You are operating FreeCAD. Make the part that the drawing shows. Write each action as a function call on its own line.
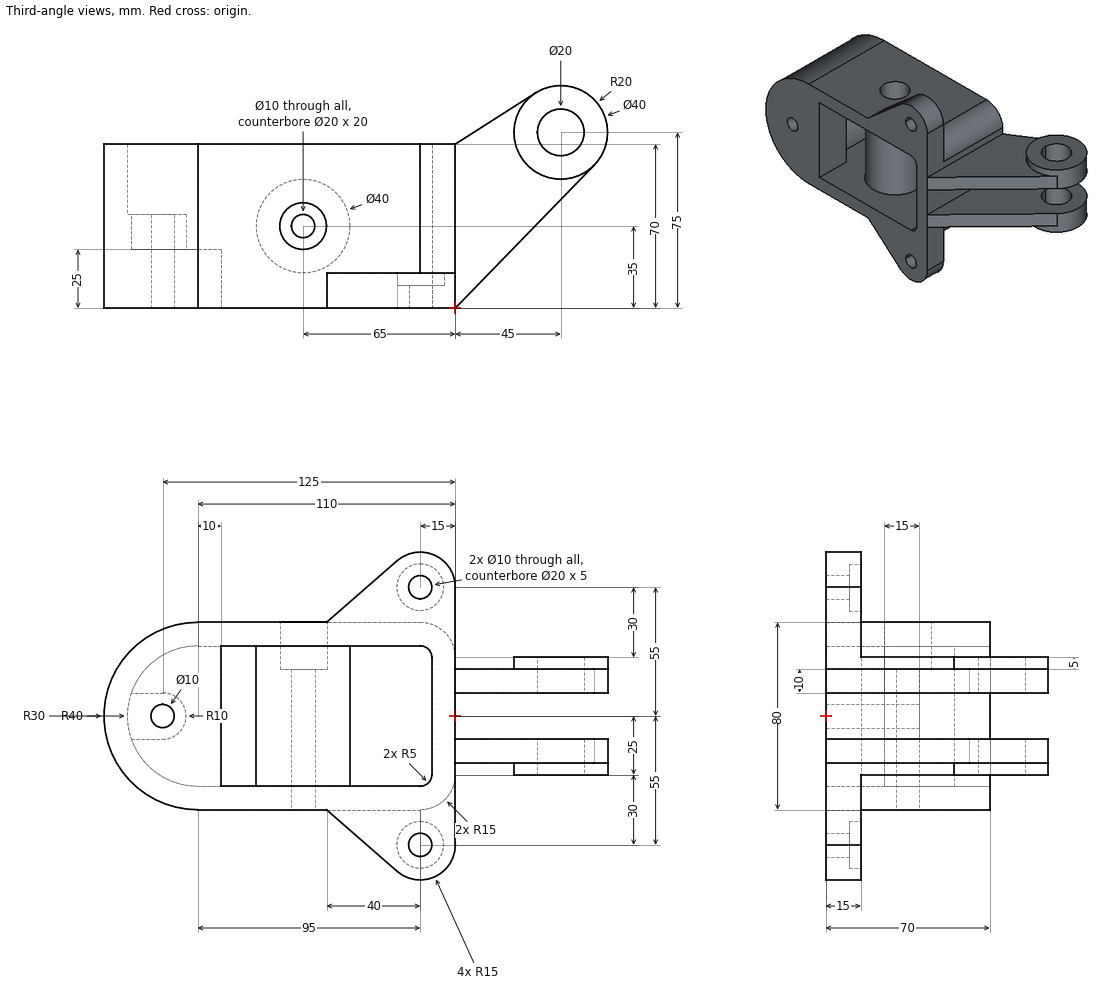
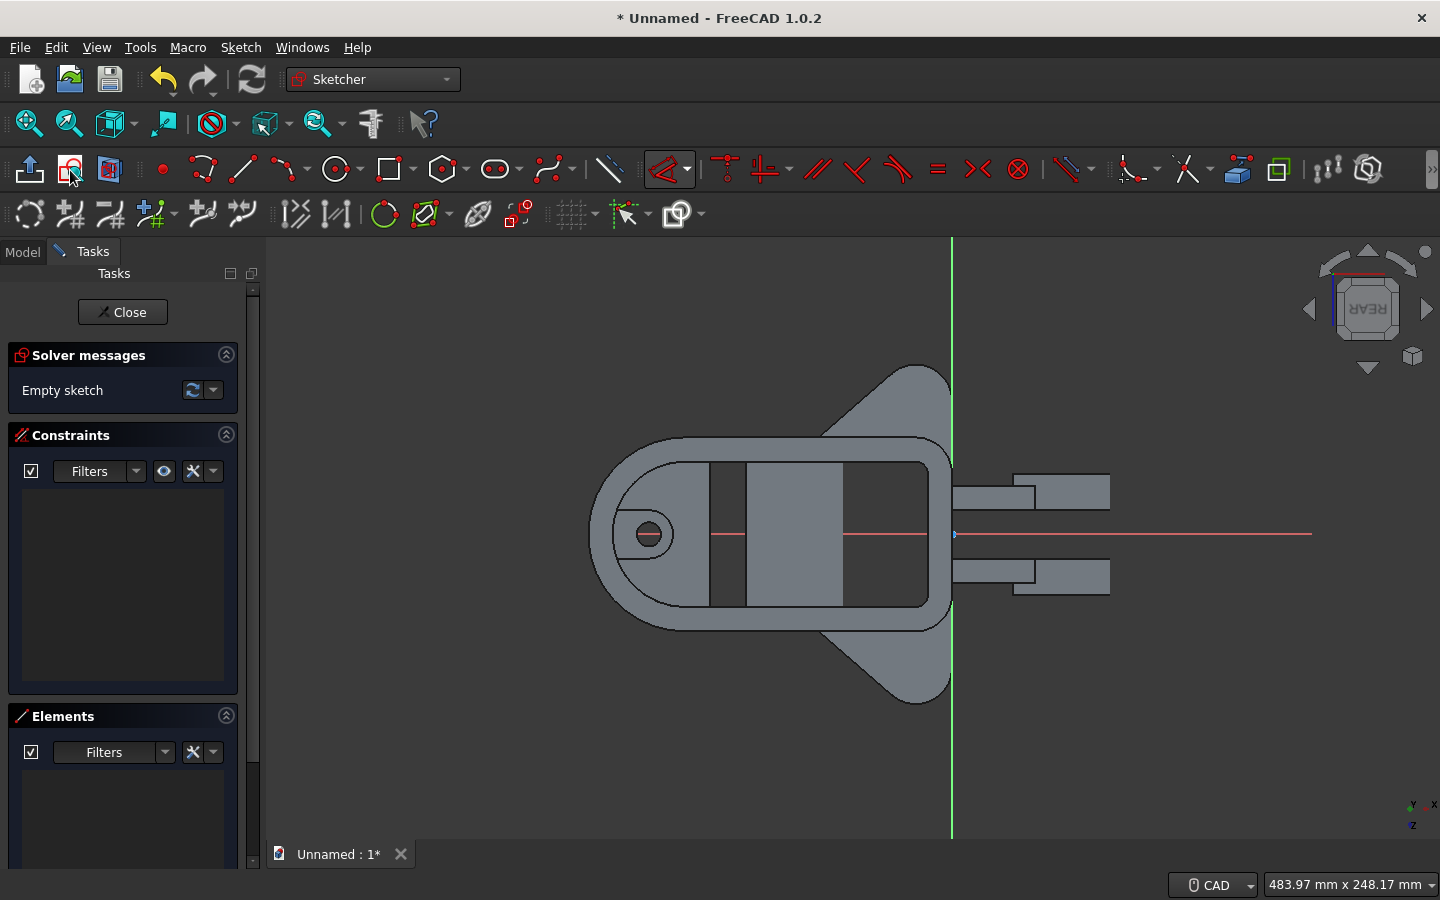
key(q)
key(s)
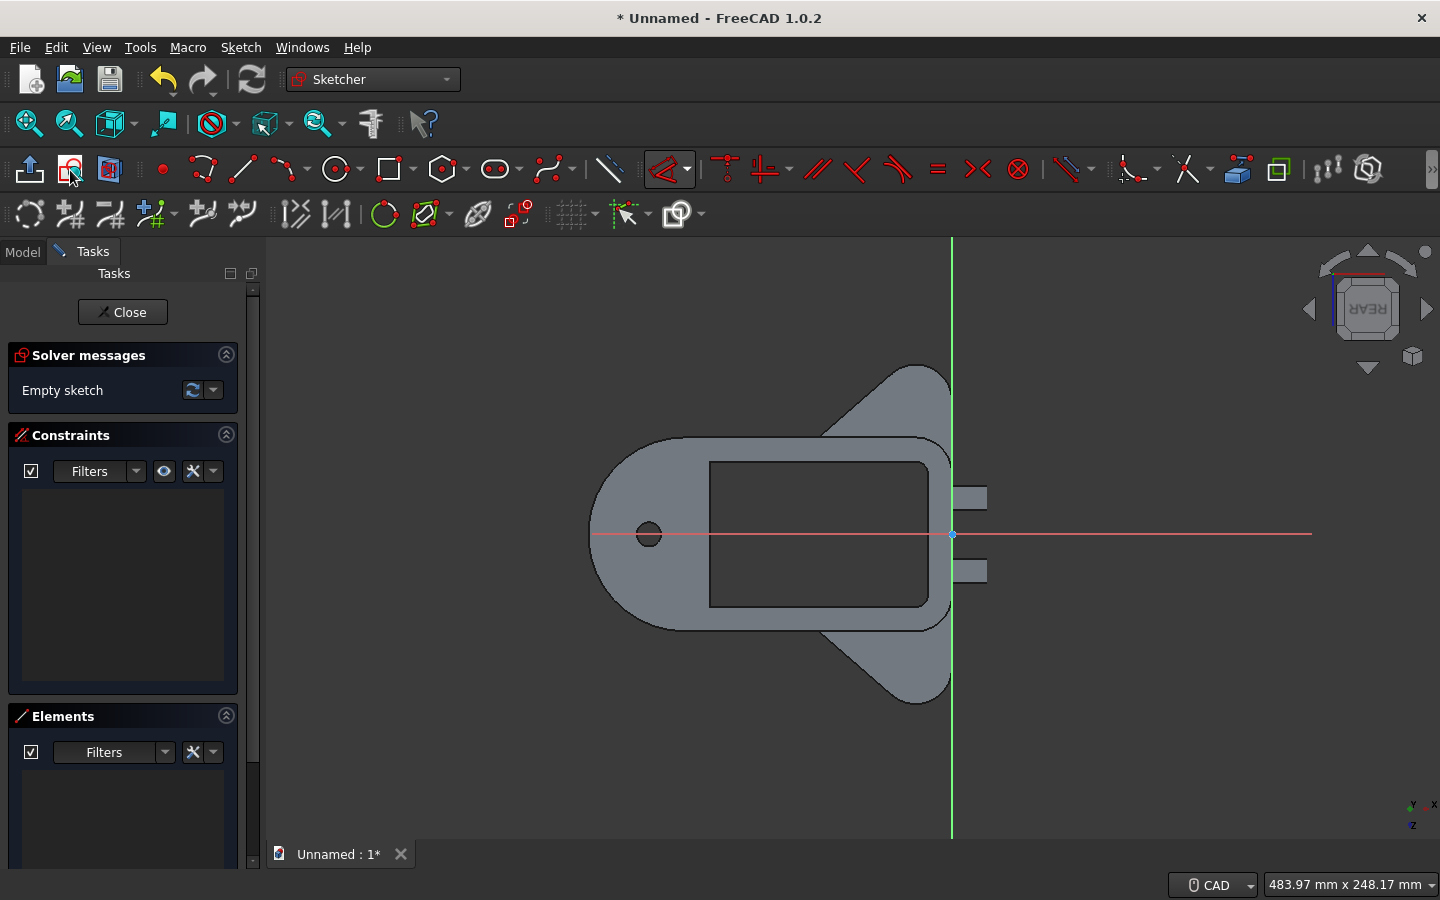
key(g)
key(c)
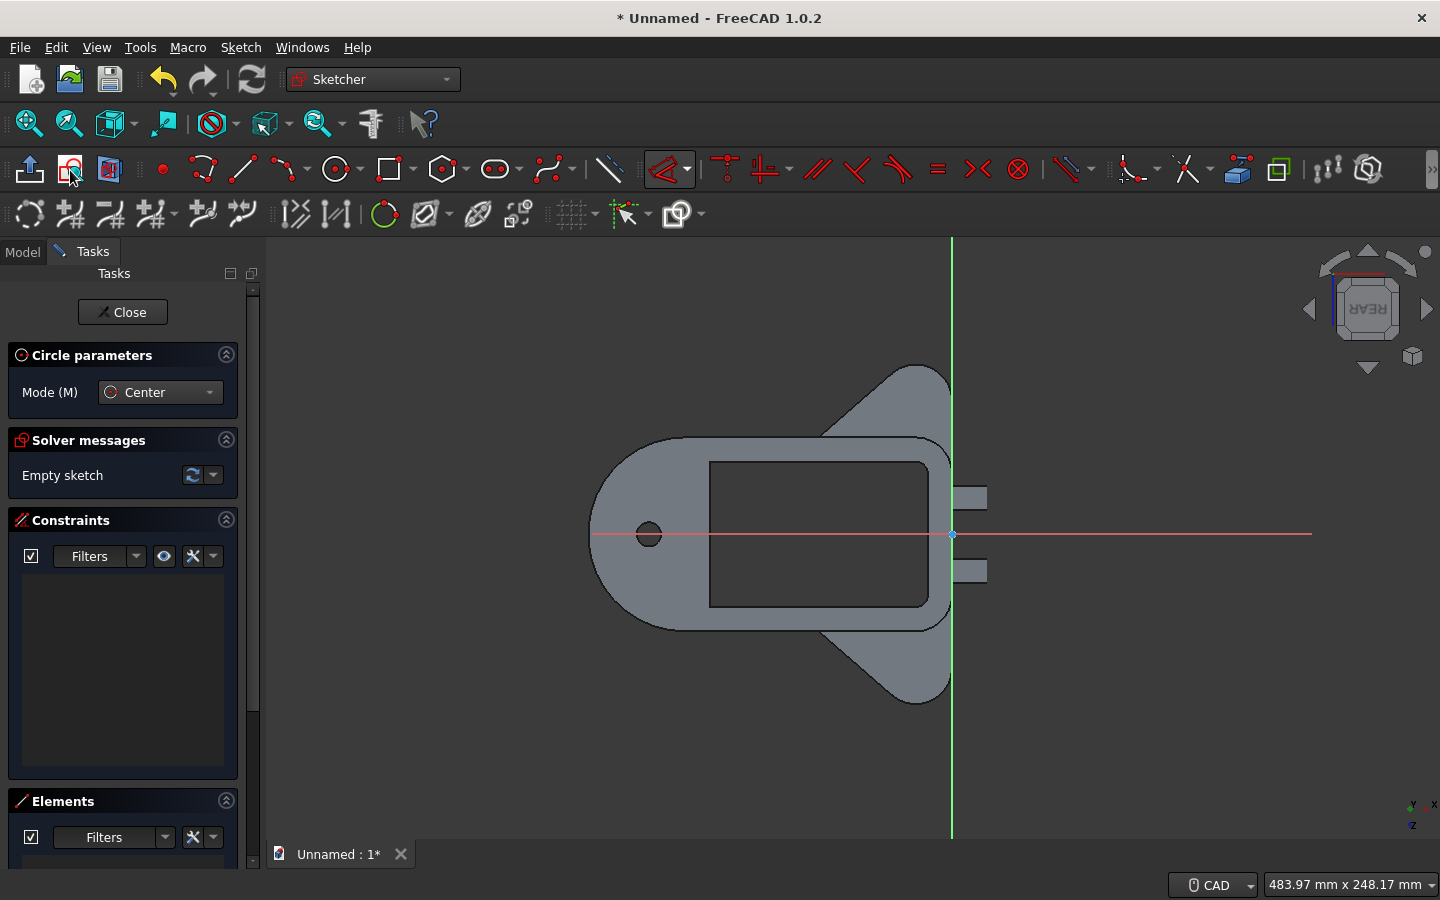
scroll(916, 668, up, 4)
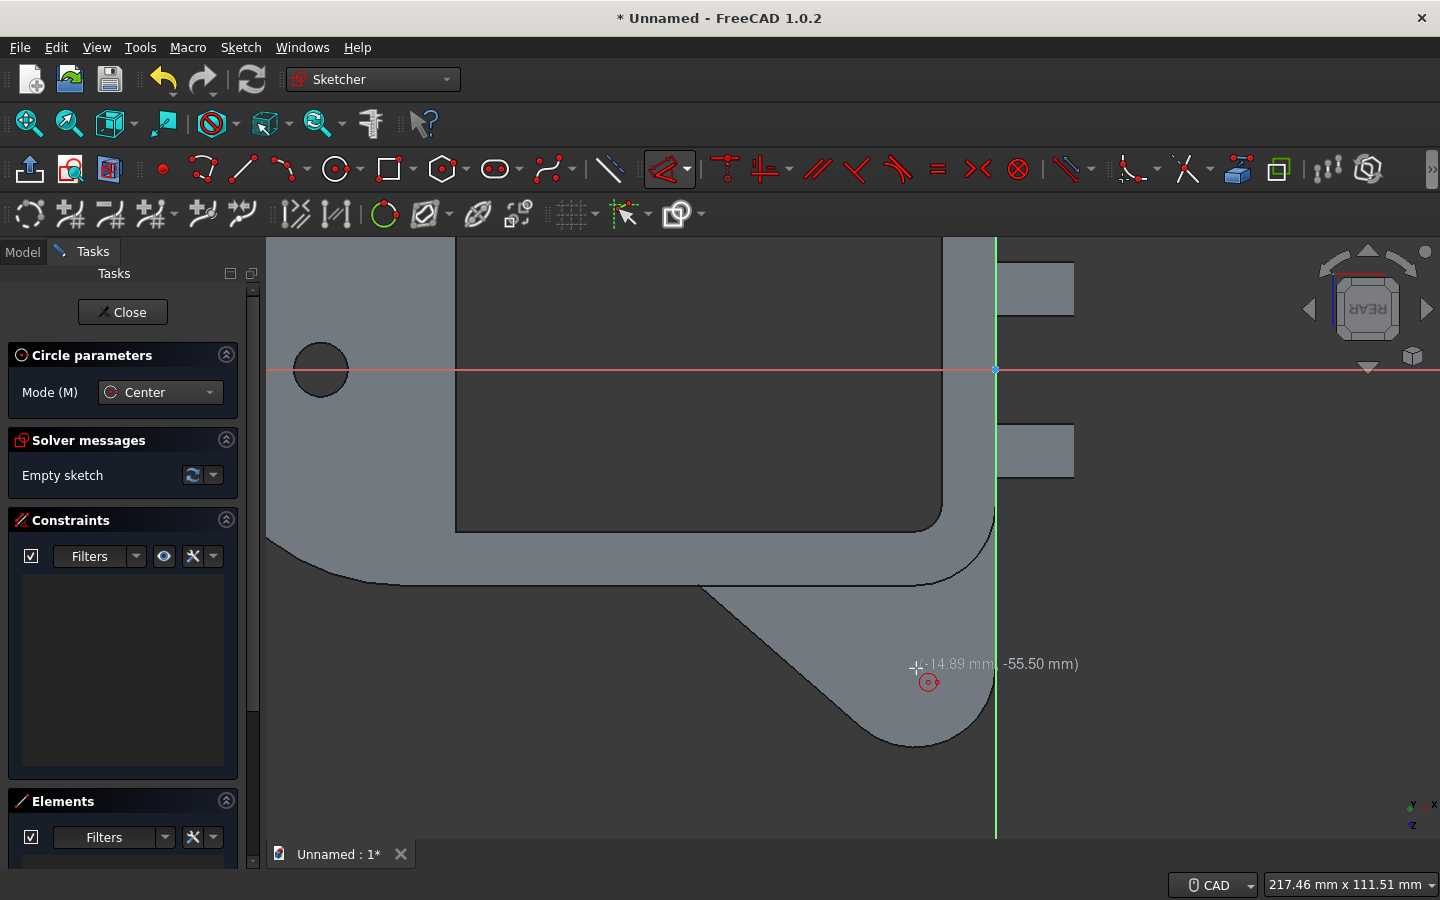
click(915, 667)
move(934, 648)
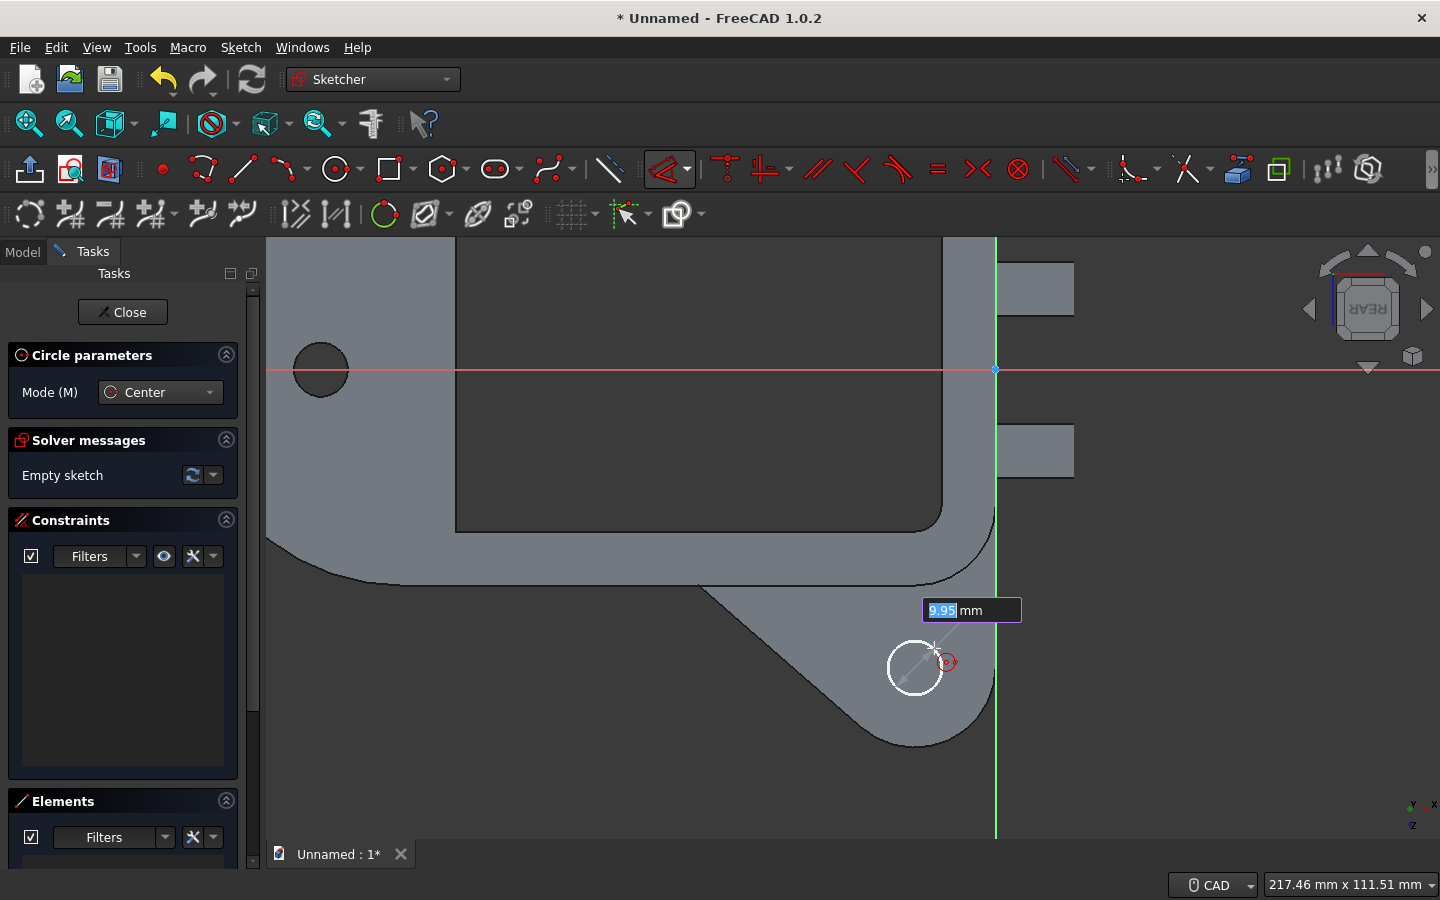
text(10)
key(Return)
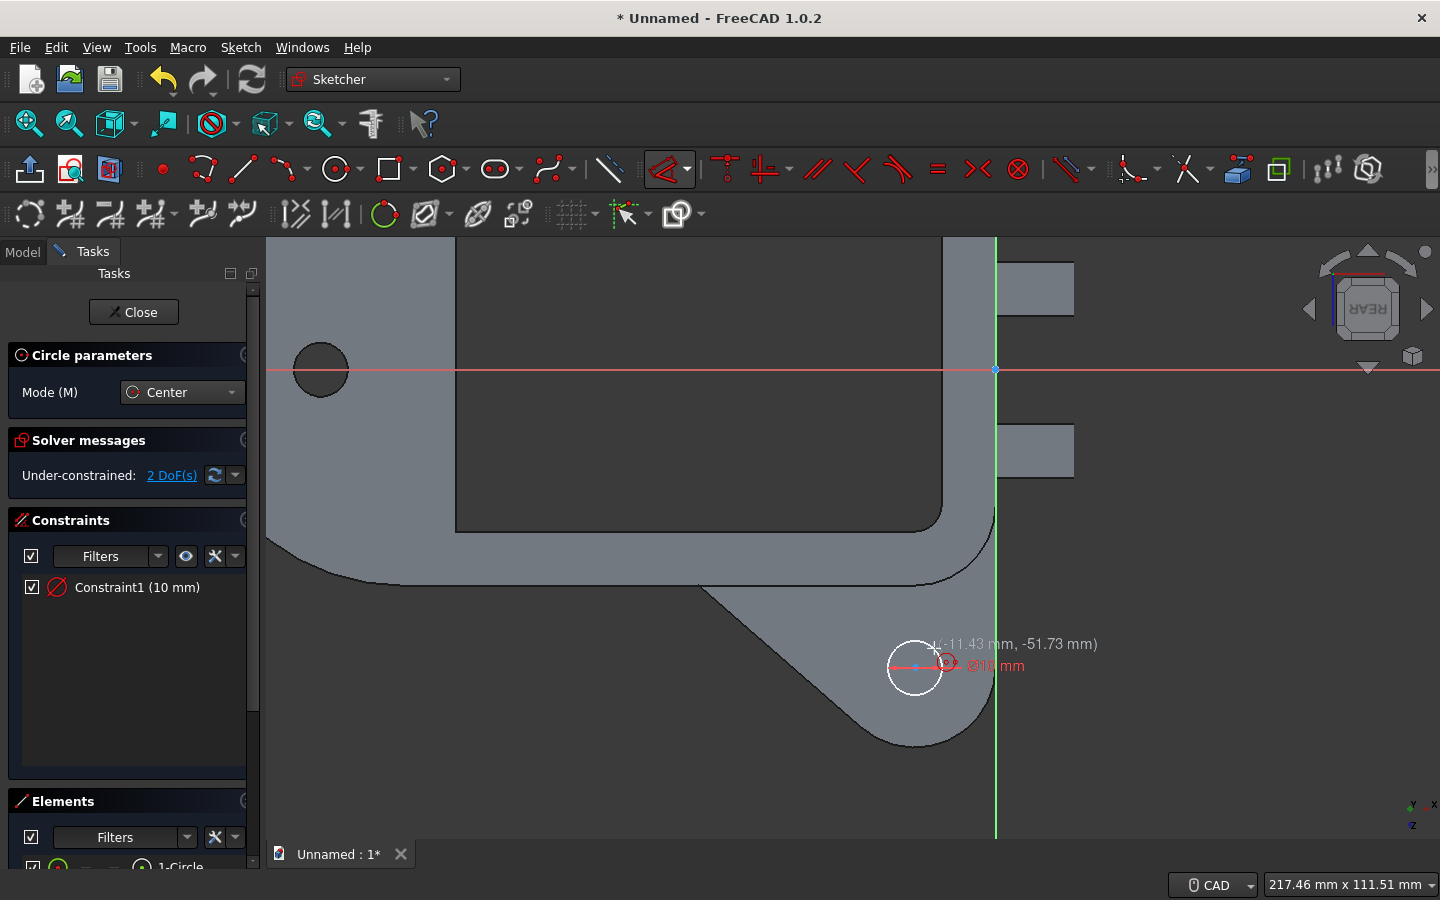
scroll(593, 743, down, 3)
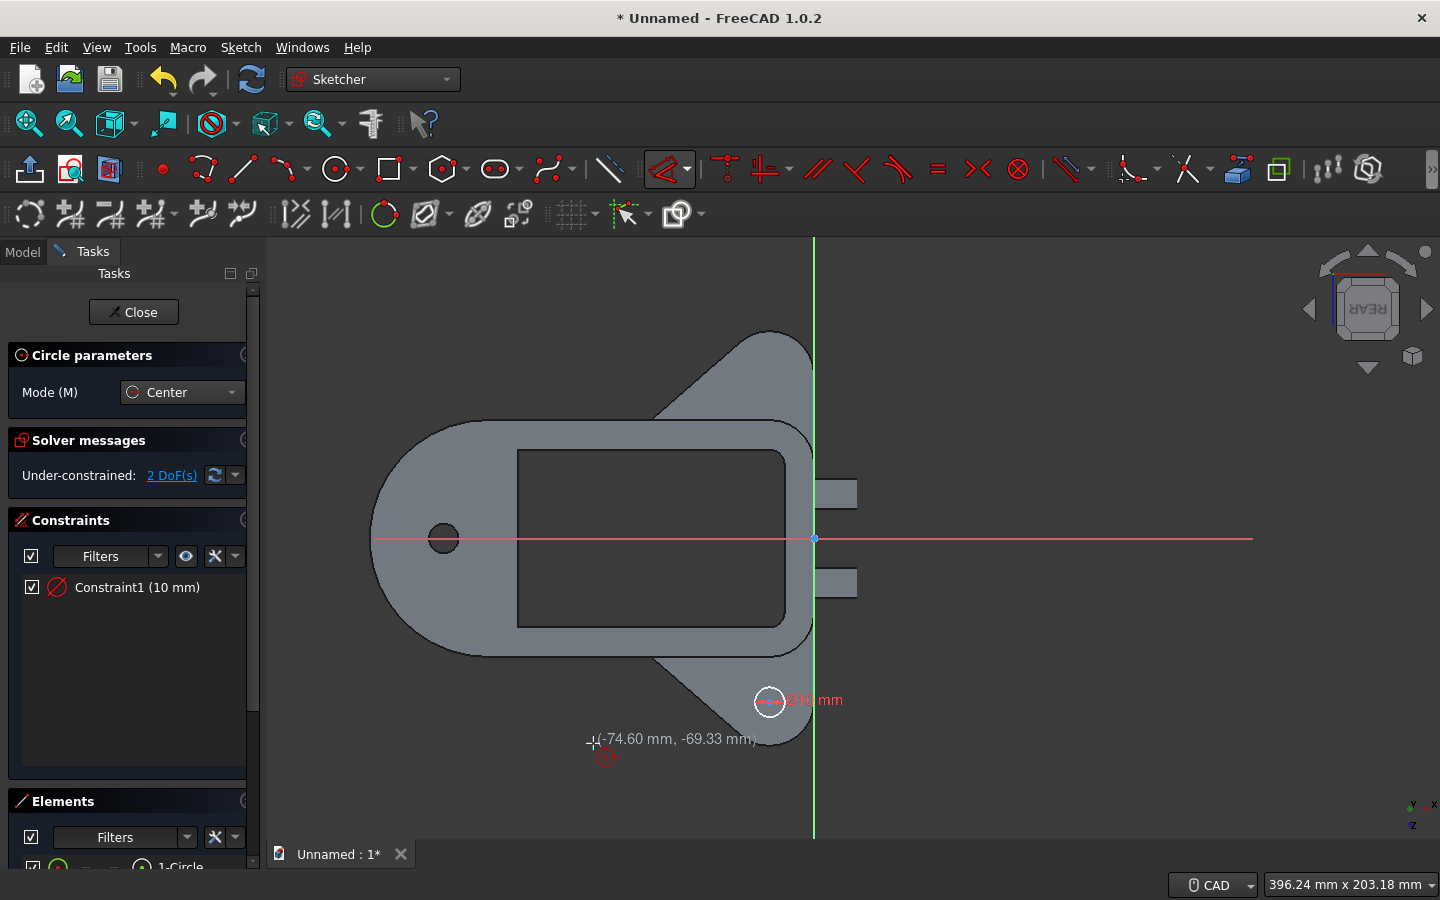
scroll(770, 376, up, 3)